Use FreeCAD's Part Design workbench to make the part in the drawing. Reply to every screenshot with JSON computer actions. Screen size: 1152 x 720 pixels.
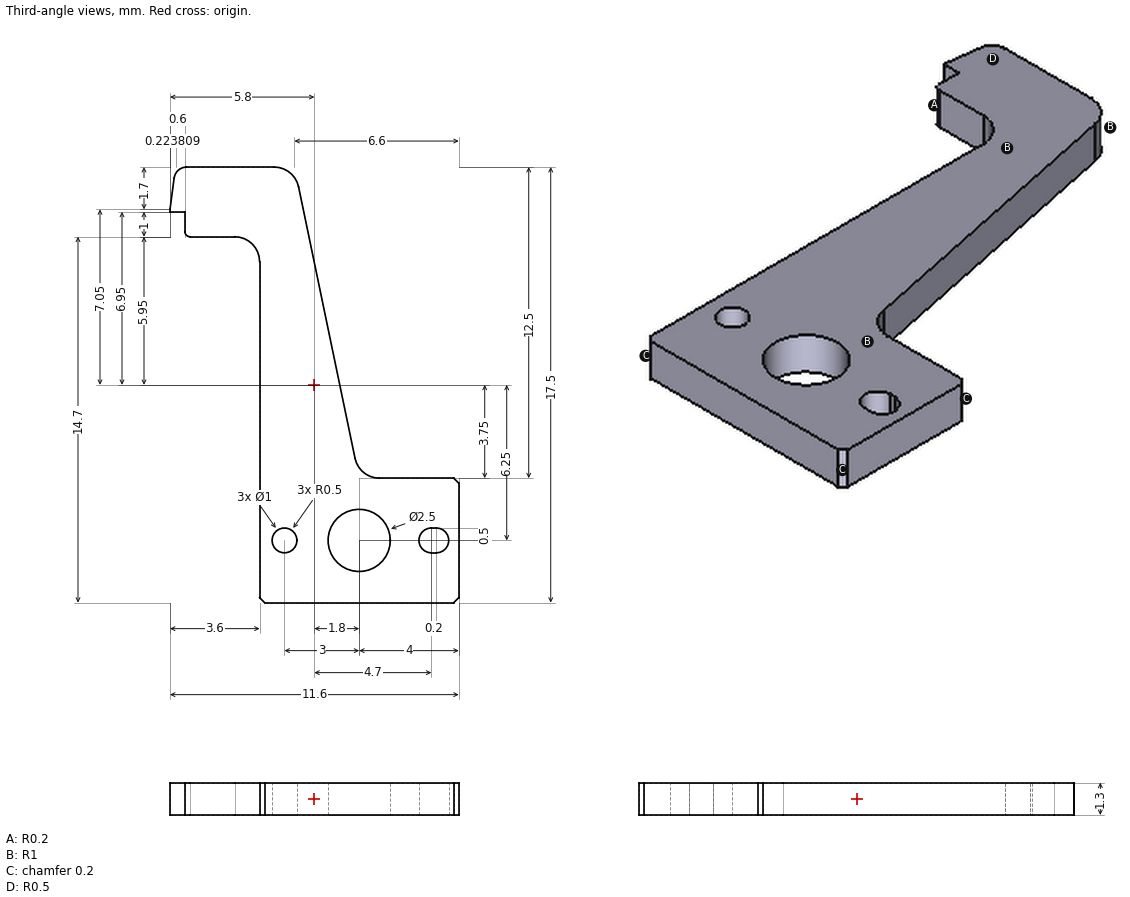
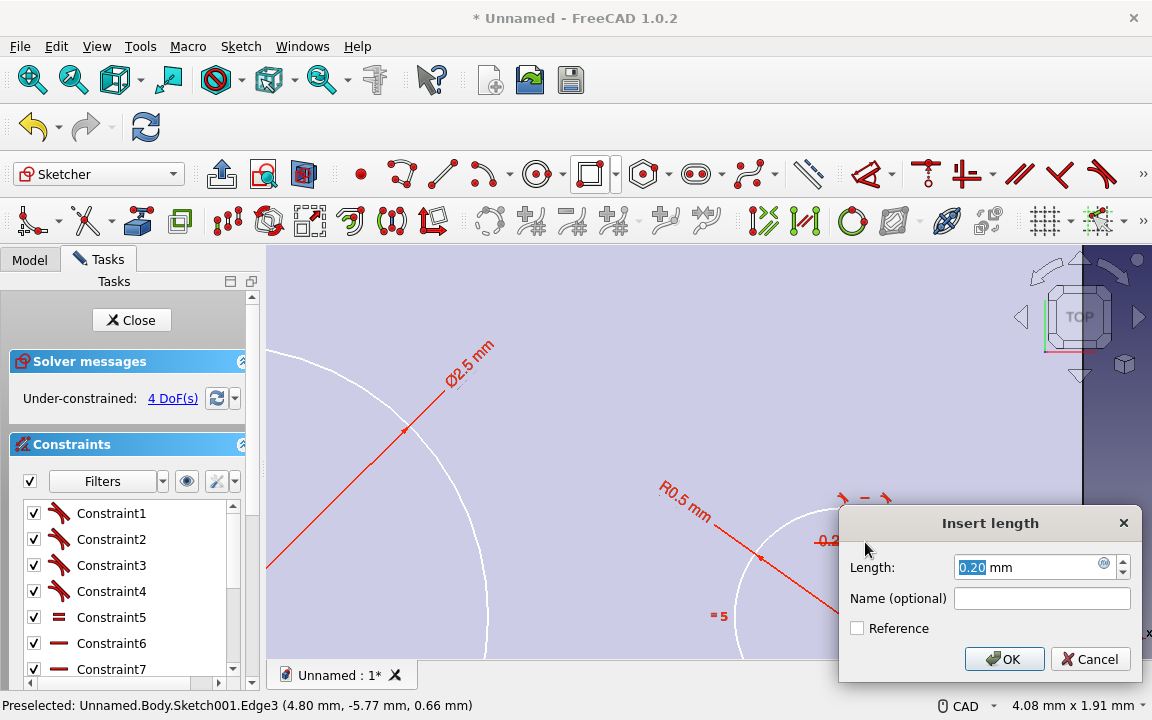
{"action": "type", "text": "0.2"}
{"action": "key", "text": "Return"}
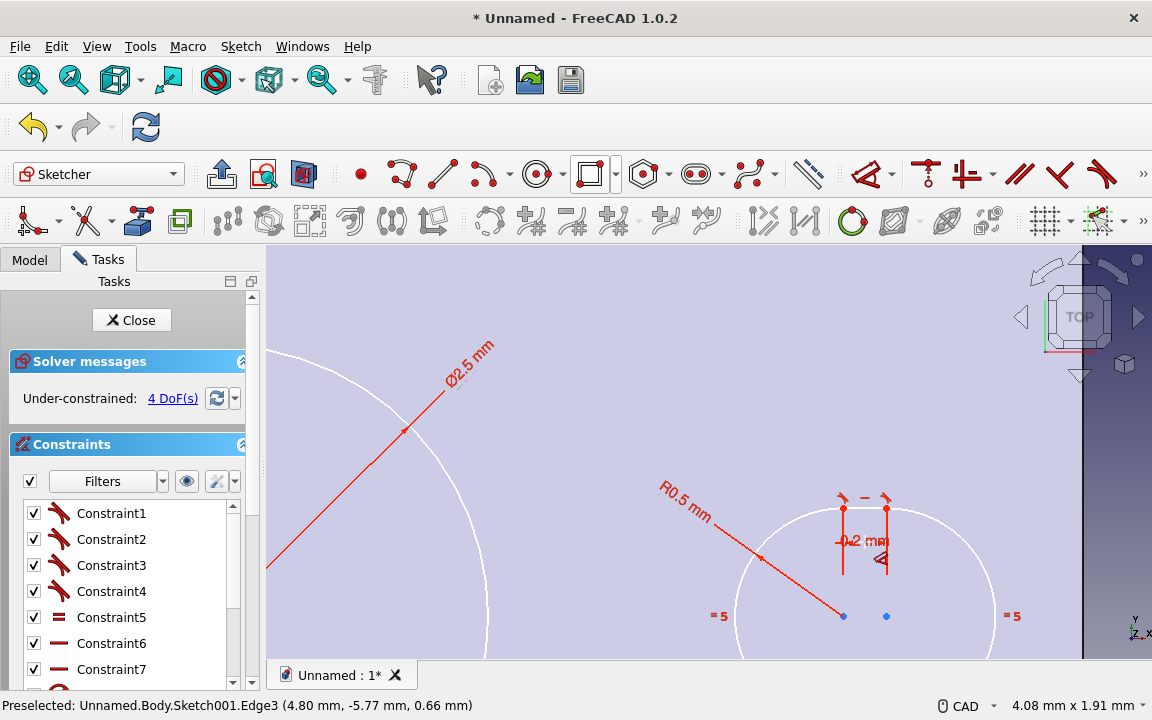
{"action": "scroll", "coordinate": [723, 528], "scroll_direction": "down", "scroll_amount": 9}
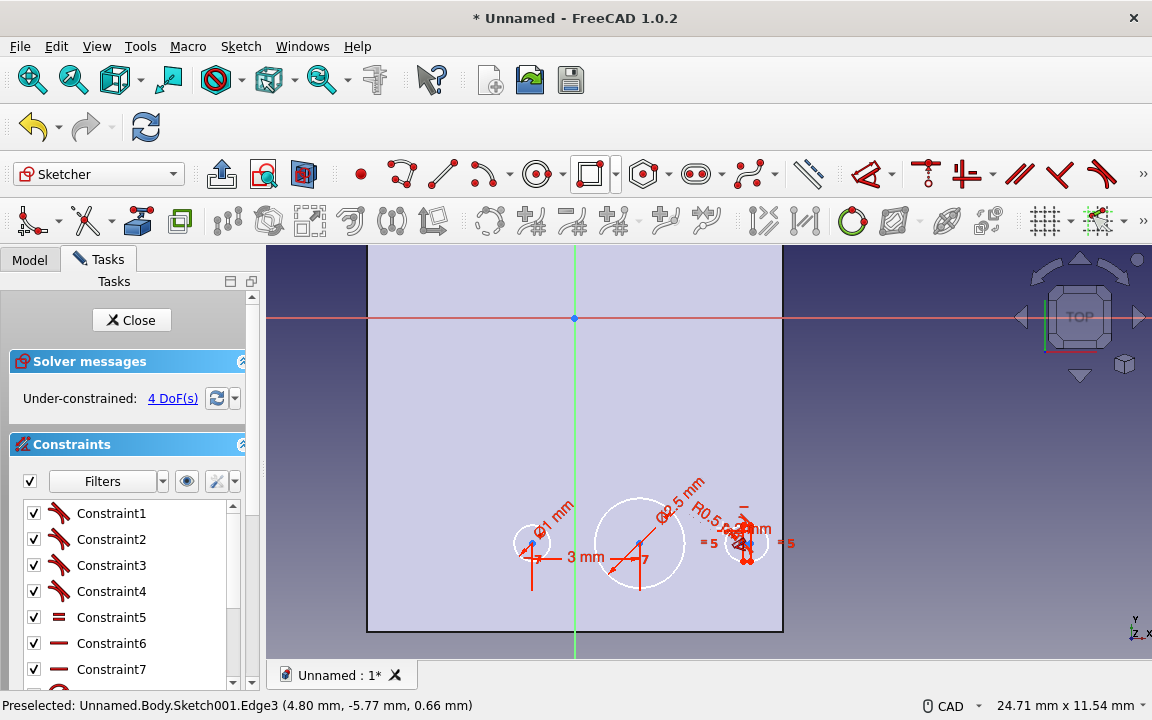
{"action": "left_click", "coordinate": [640, 543]}
{"action": "left_click", "coordinate": [607, 284]}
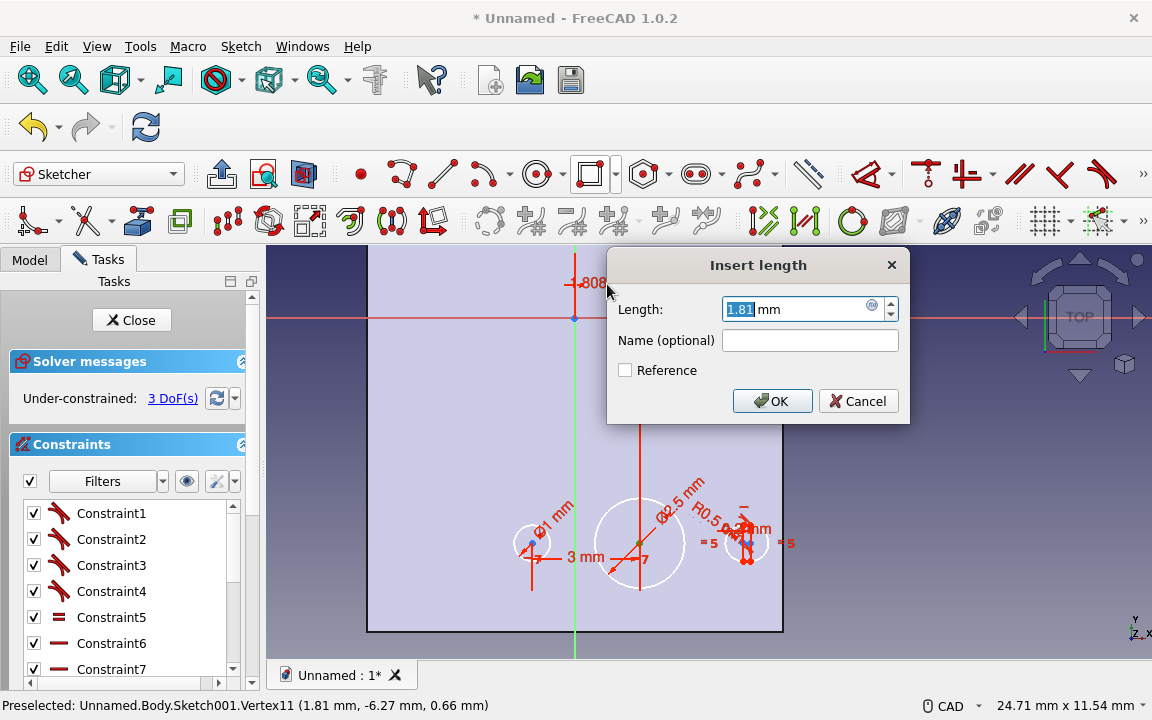
{"action": "type", "text": "1.8"}
{"action": "key", "text": "Return"}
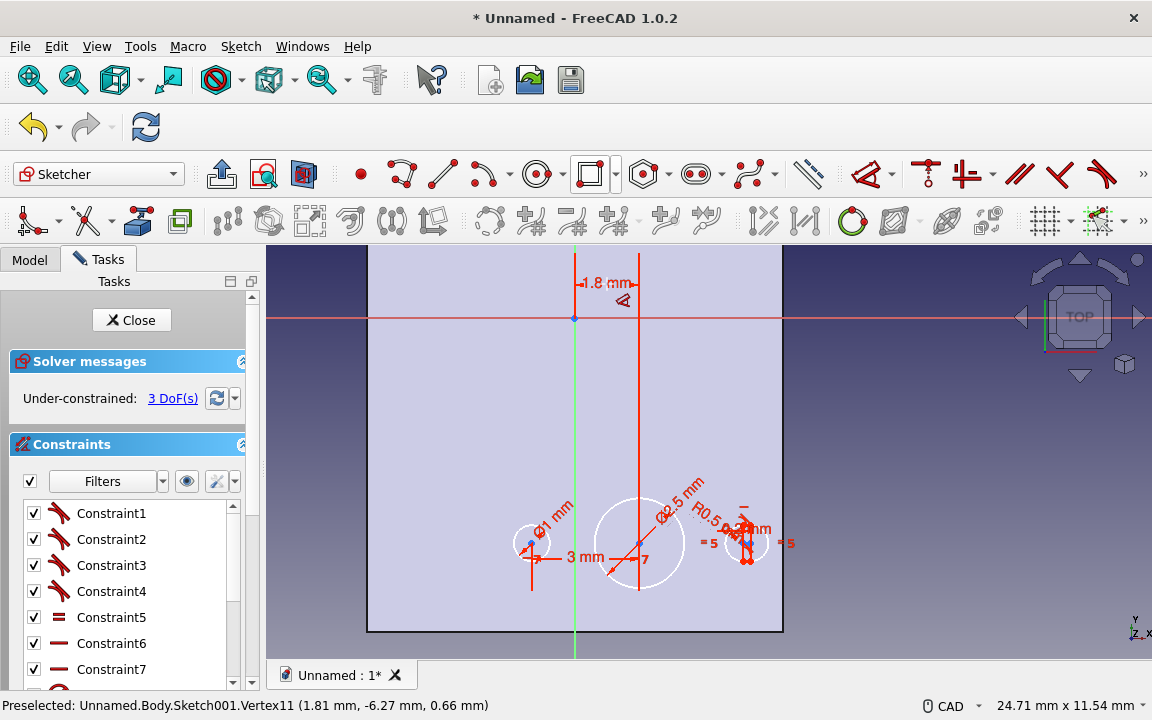
{"action": "scroll", "coordinate": [743, 525], "scroll_direction": "up", "scroll_amount": 3}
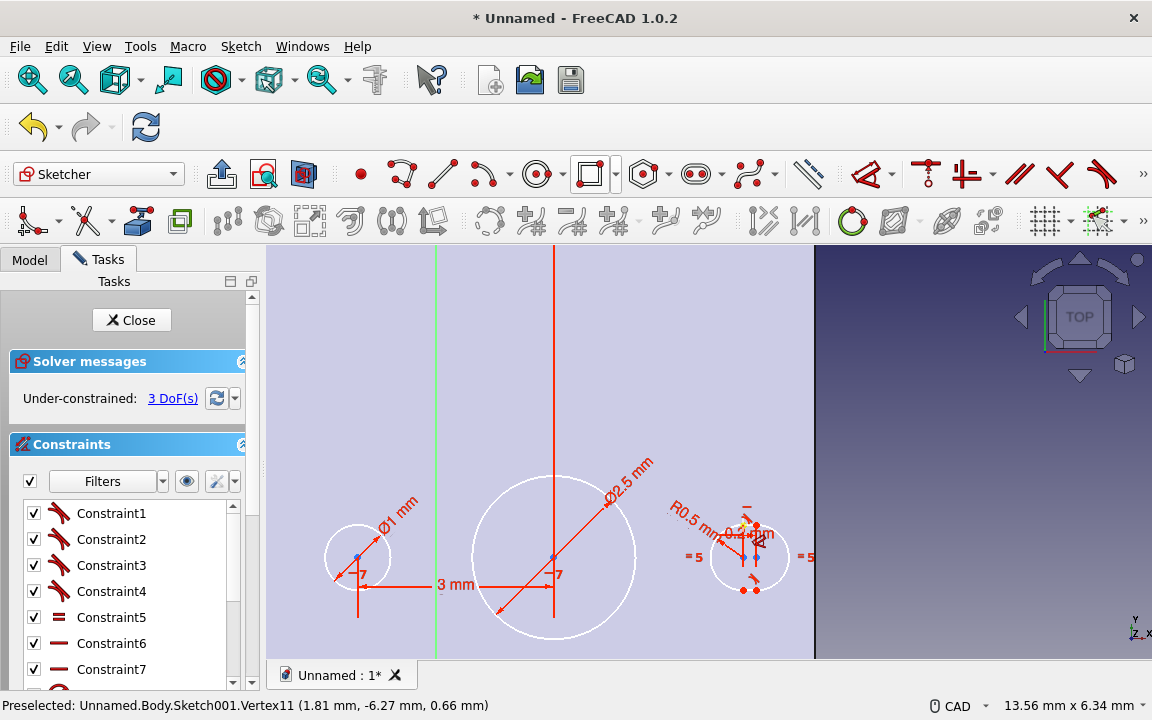
{"action": "left_click", "coordinate": [743, 525]}
{"action": "left_click", "coordinate": [590, 559]}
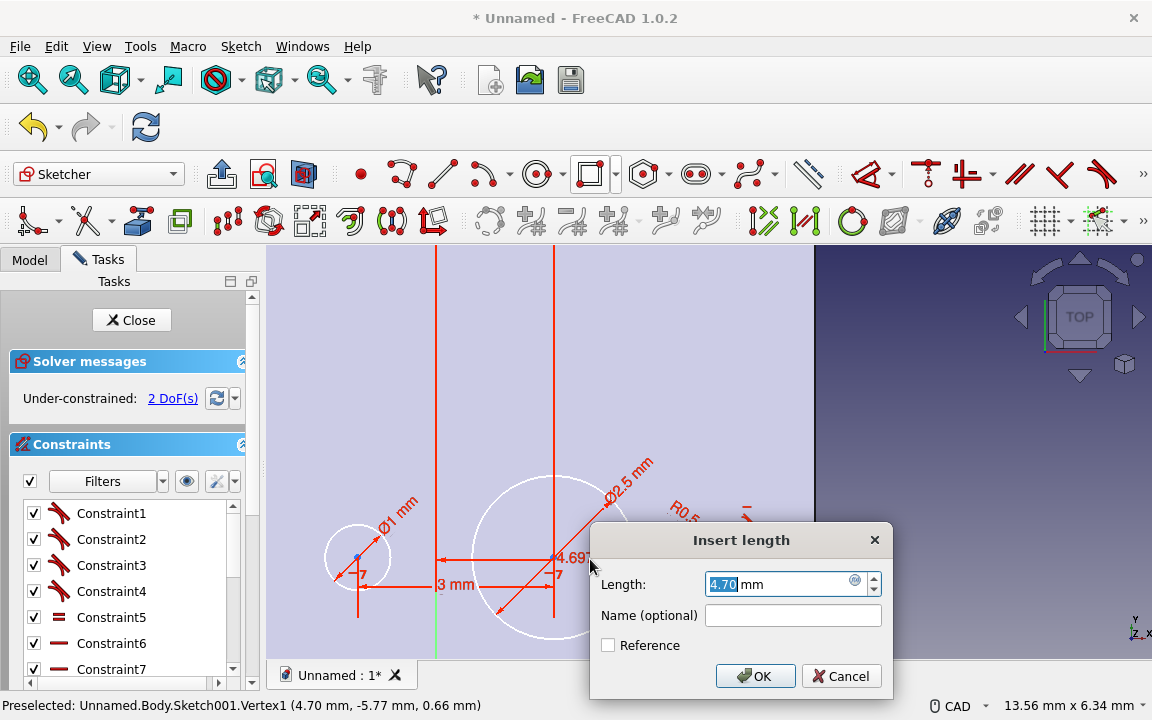
{"action": "type", "text": "4.7"}
{"action": "key", "text": "Return"}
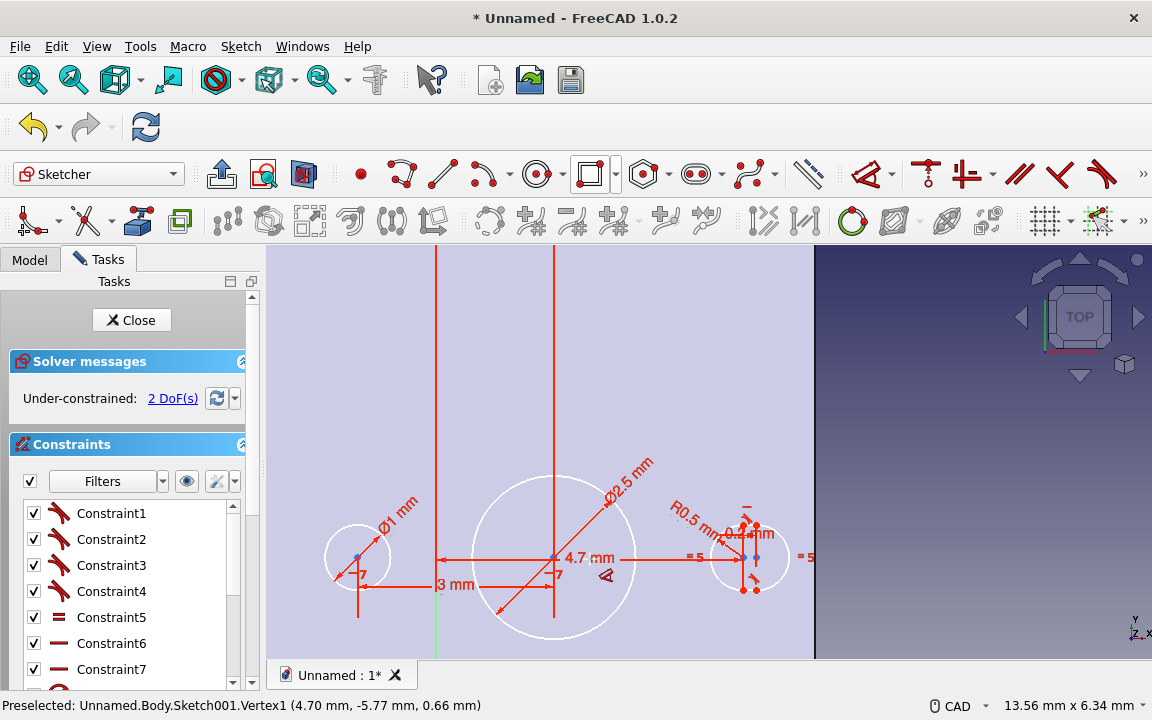
{"action": "left_click", "coordinate": [554, 558]}
{"action": "left_click", "coordinate": [402, 415]}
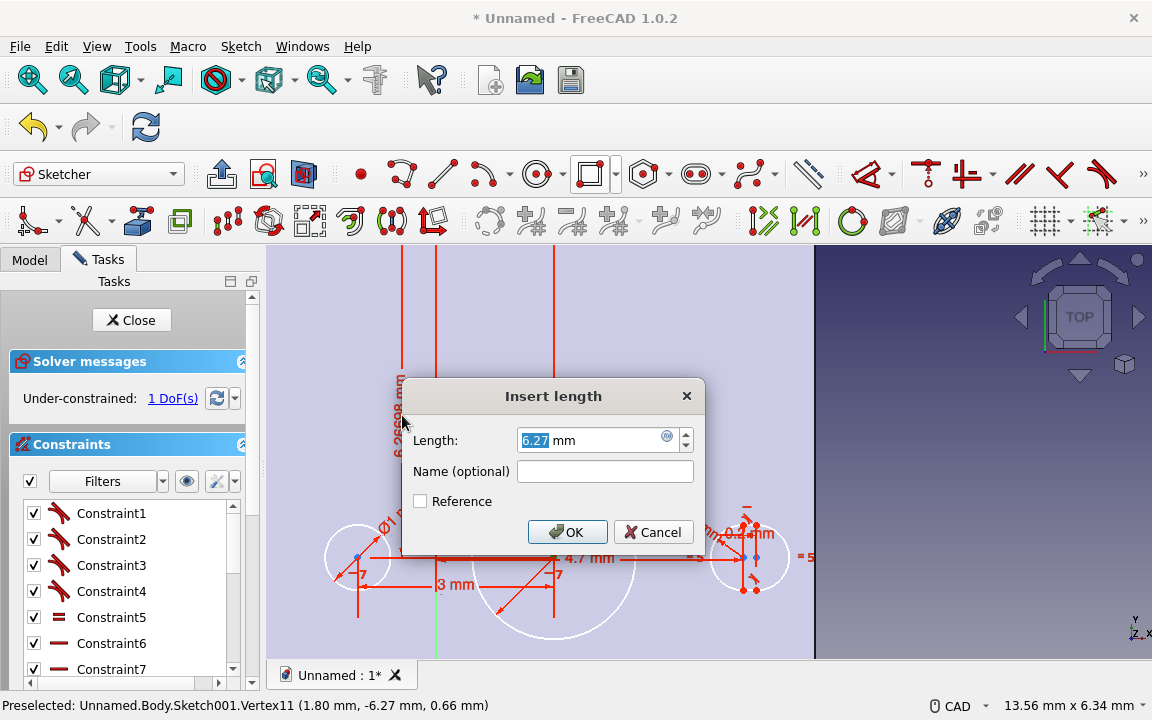
{"action": "type", "text": "6.25"}
{"action": "key", "text": "Return"}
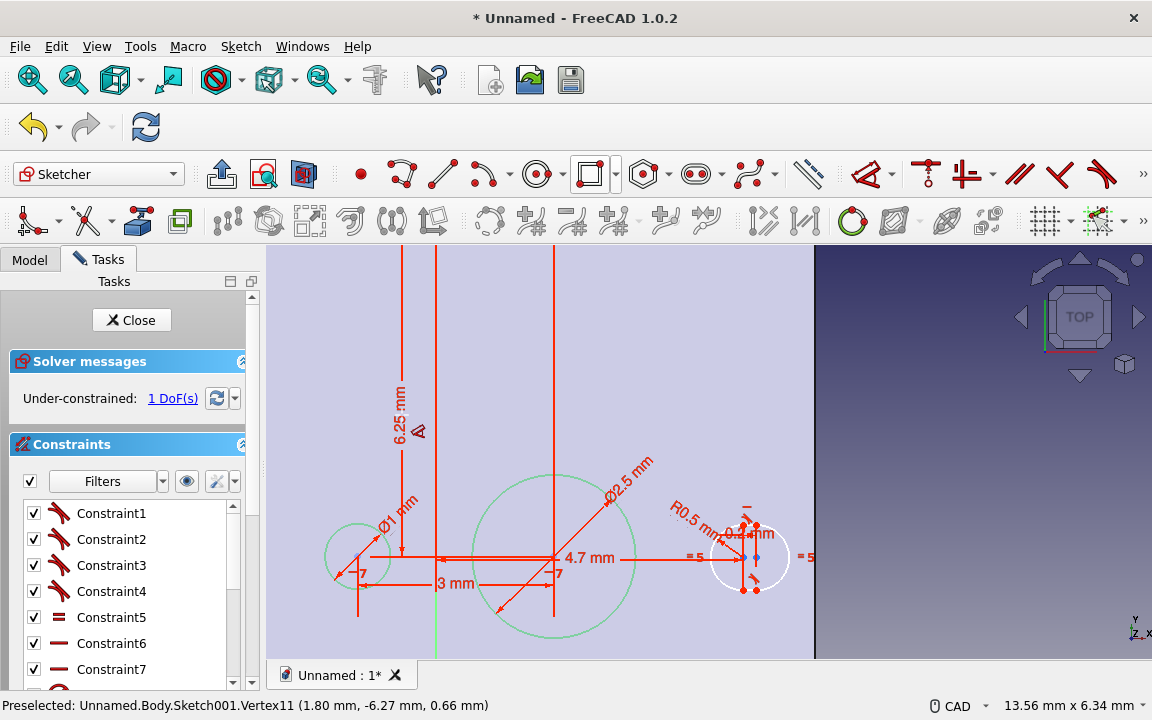
{"action": "left_click", "coordinate": [743, 525]}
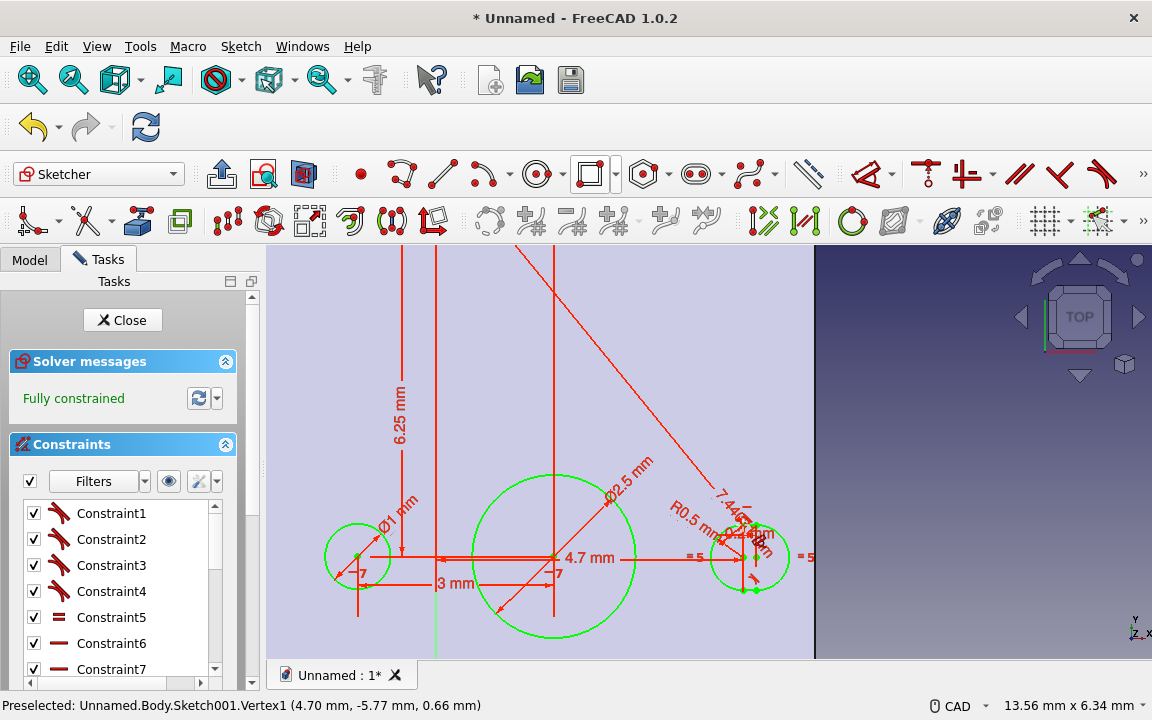
{"action": "left_click", "coordinate": [554, 557]}
{"action": "left_click", "coordinate": [520, 534]}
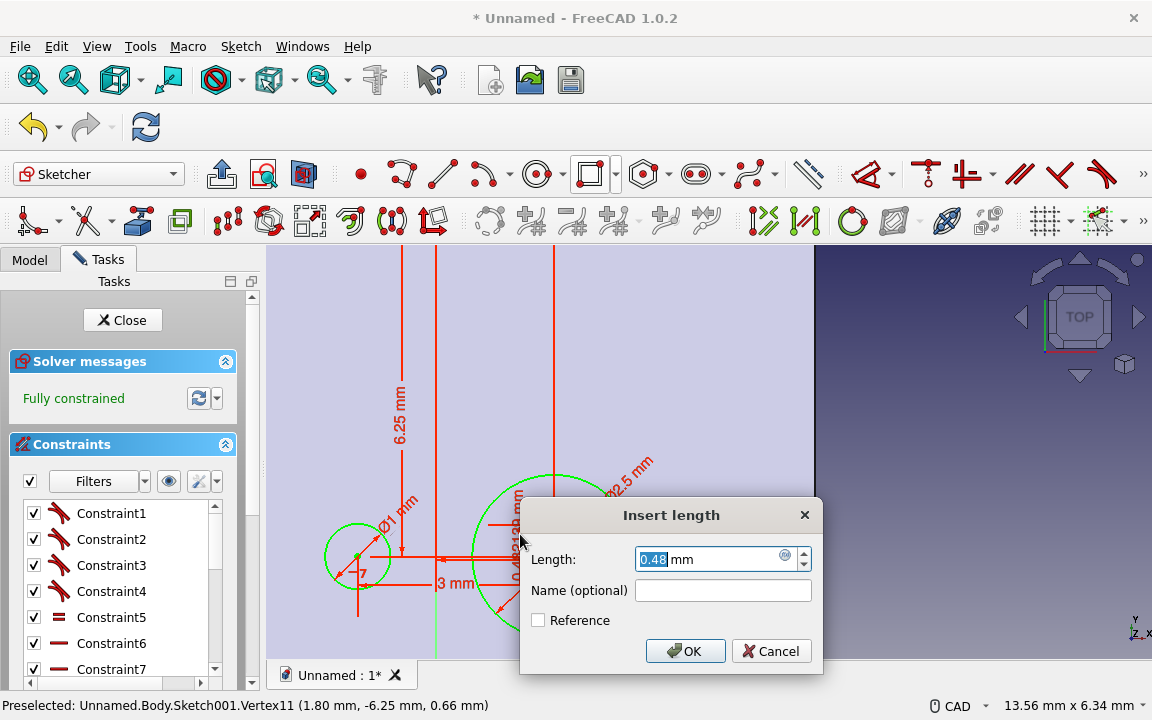
{"action": "type", "text": "0.5"}
{"action": "key", "text": "Return"}
{"action": "key", "text": "Escape"}